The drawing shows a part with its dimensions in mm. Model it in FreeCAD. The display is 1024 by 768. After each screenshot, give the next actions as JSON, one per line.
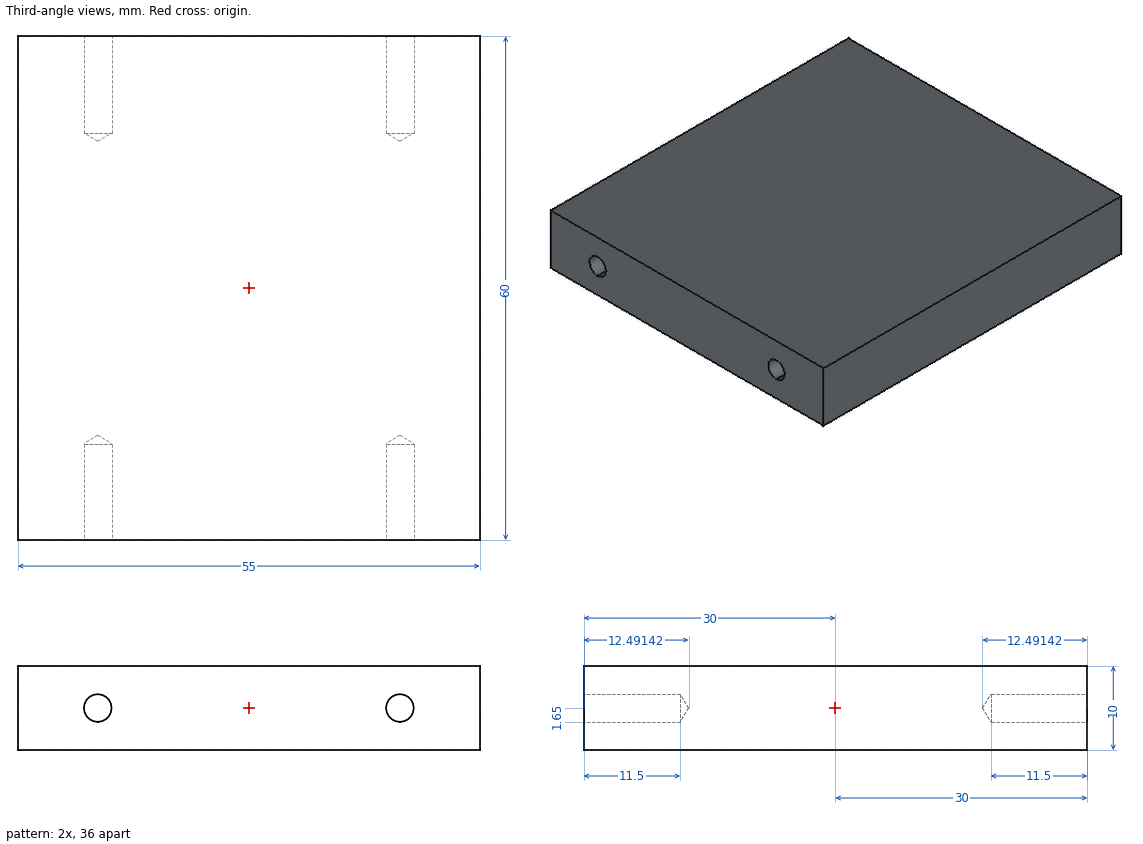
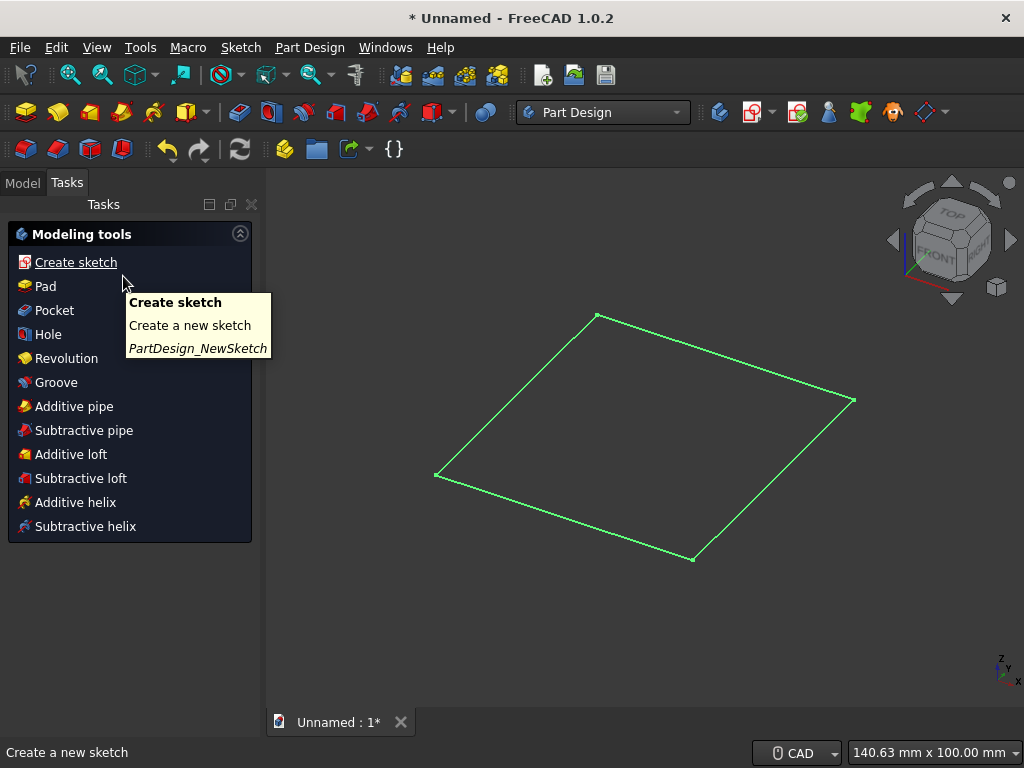
{"action": "left_click", "coordinate": [26, 112]}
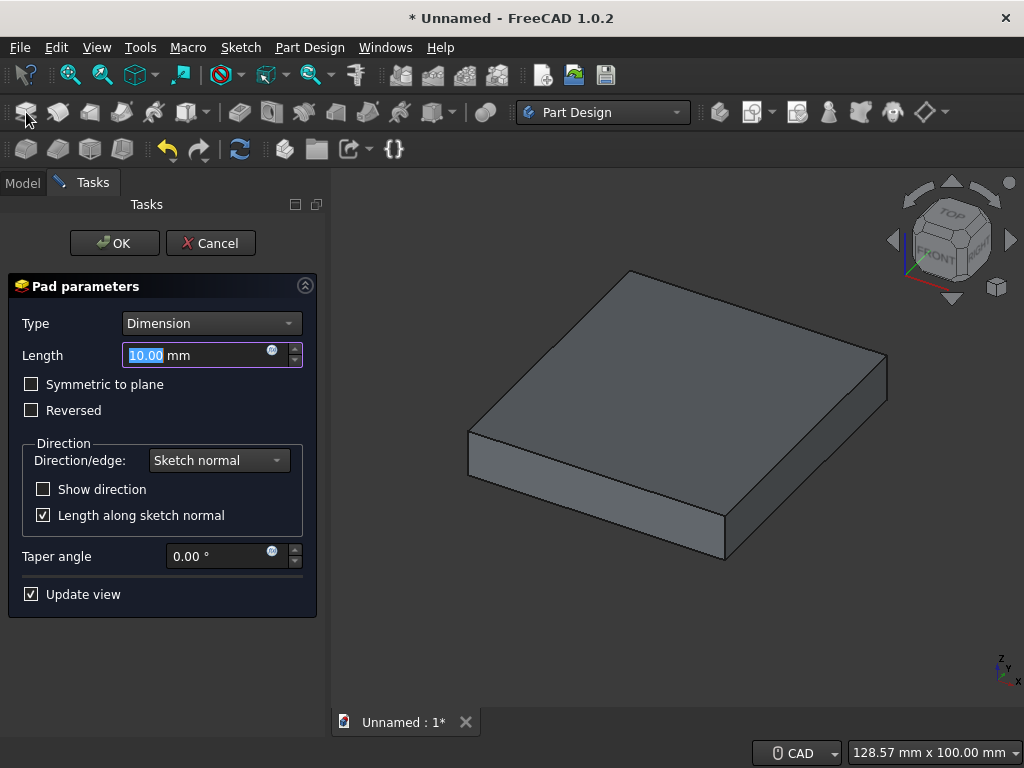
{"action": "type", "text": "10"}
{"action": "key", "text": "Tab"}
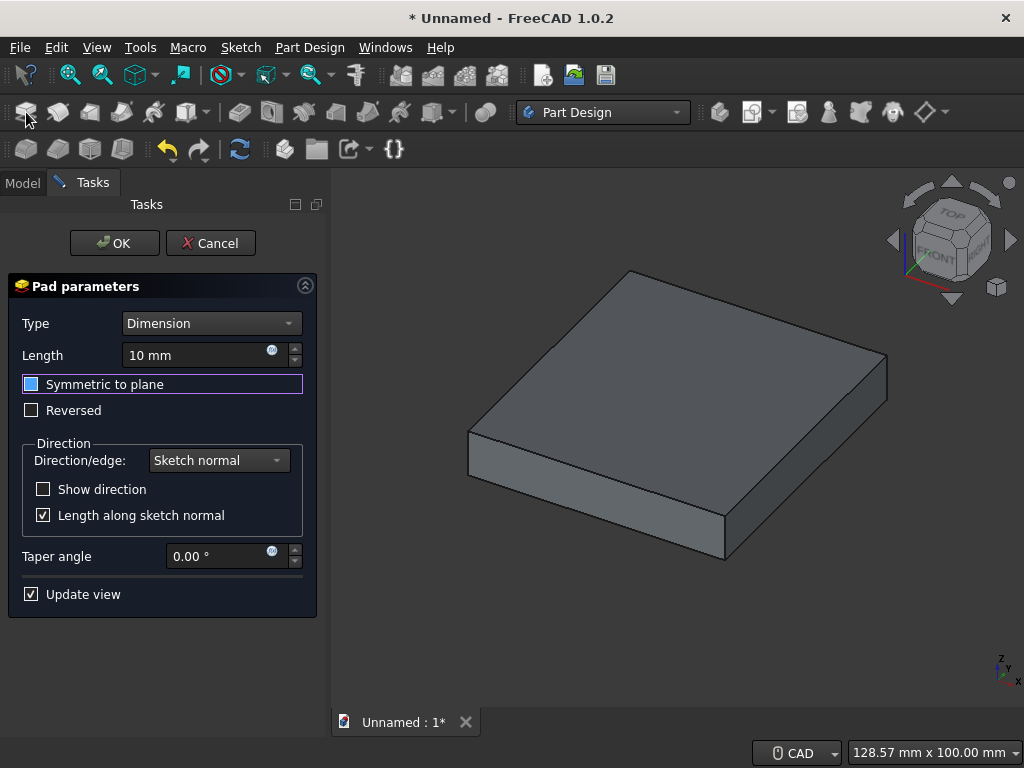
{"action": "left_click", "coordinate": [30, 384]}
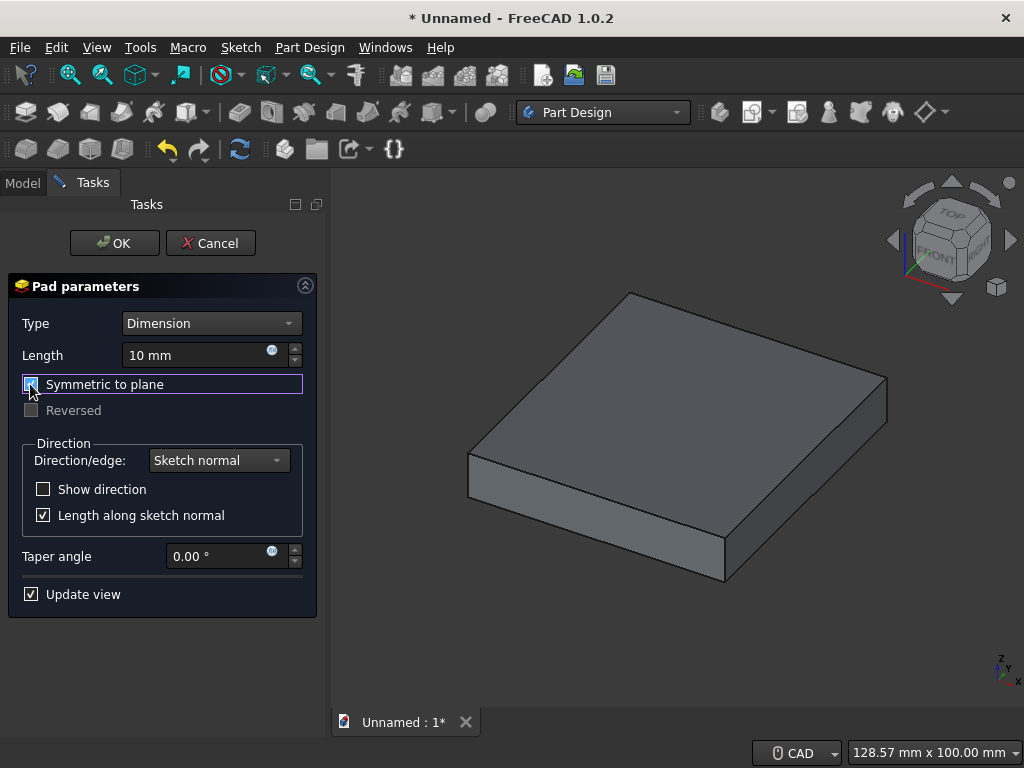
{"action": "left_click", "coordinate": [115, 243]}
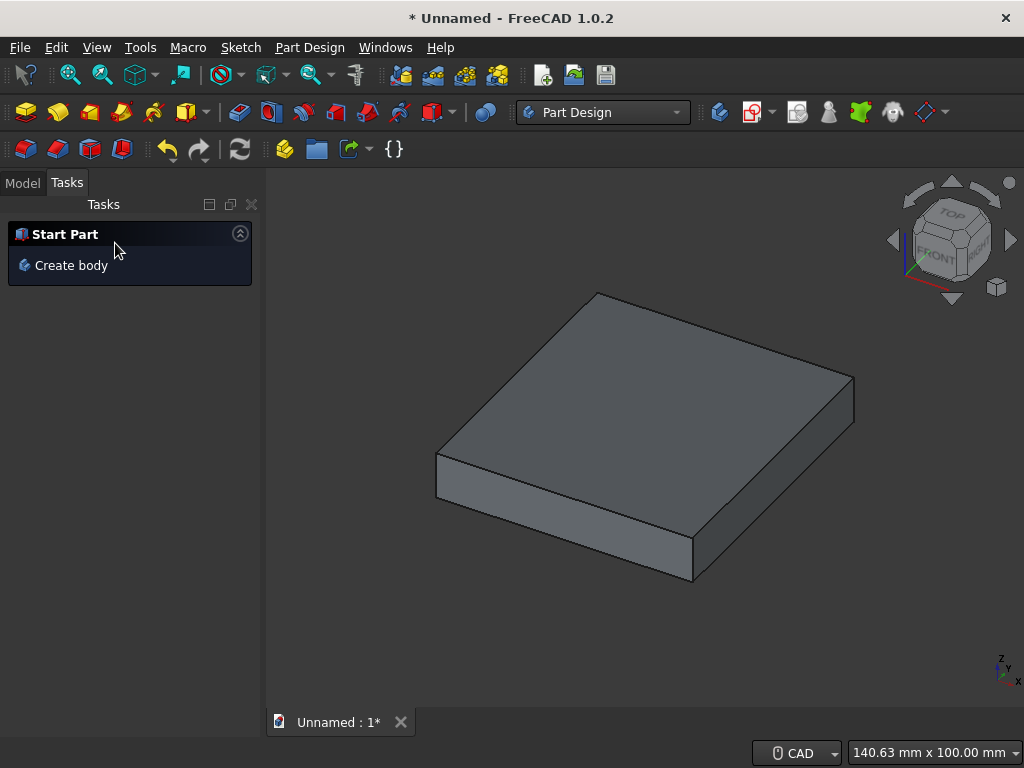
{"action": "left_click", "coordinate": [23, 182]}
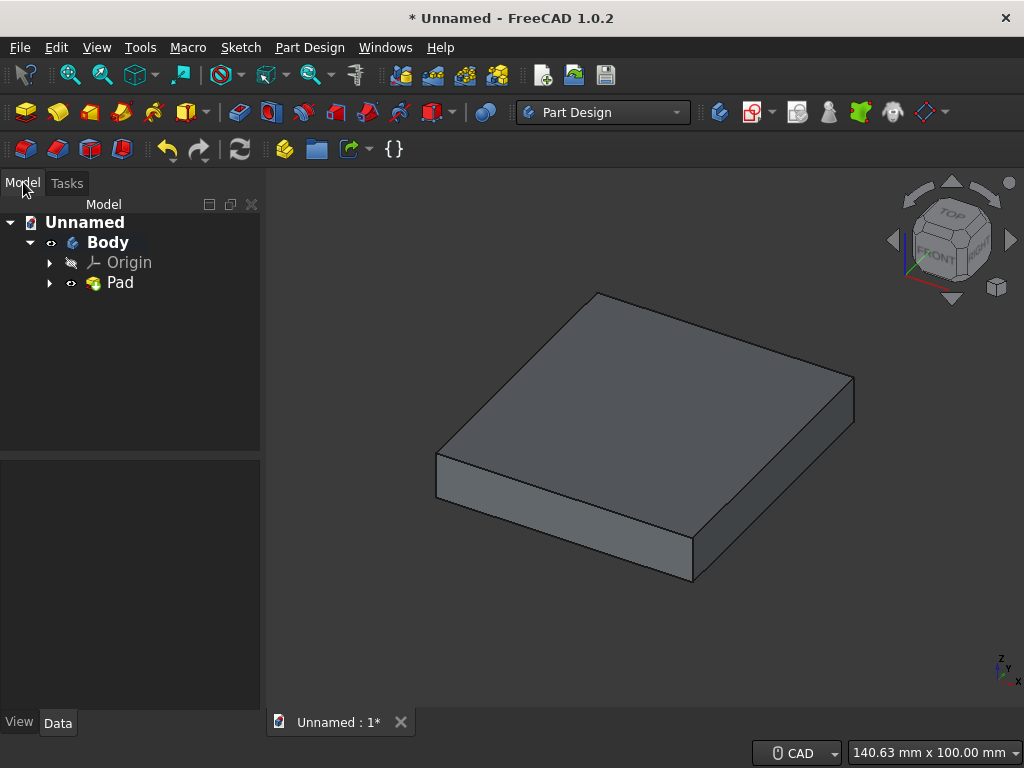
{"action": "left_click", "coordinate": [50, 263]}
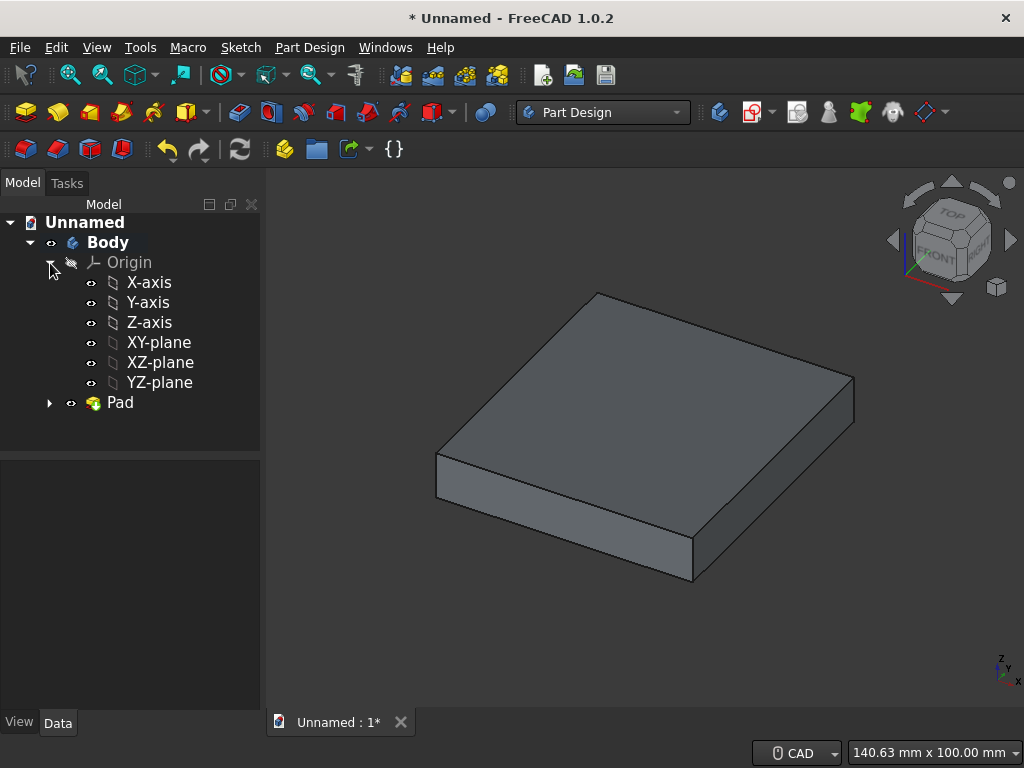
{"action": "left_click", "coordinate": [136, 383]}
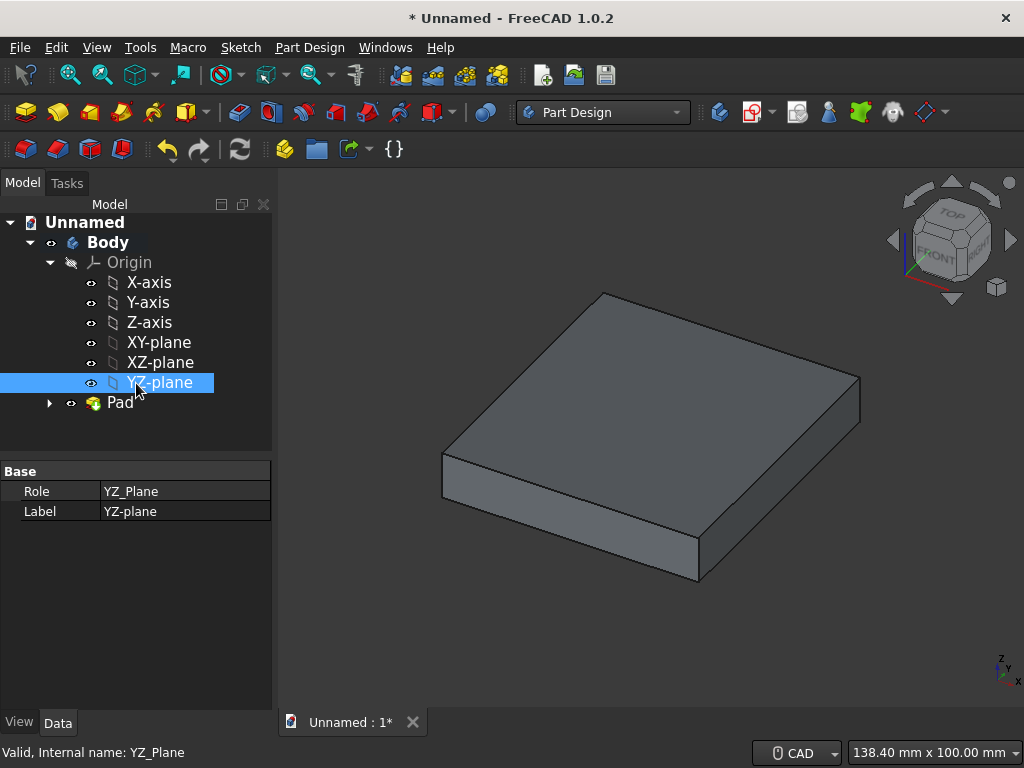
{"action": "left_click", "coordinate": [926, 112]}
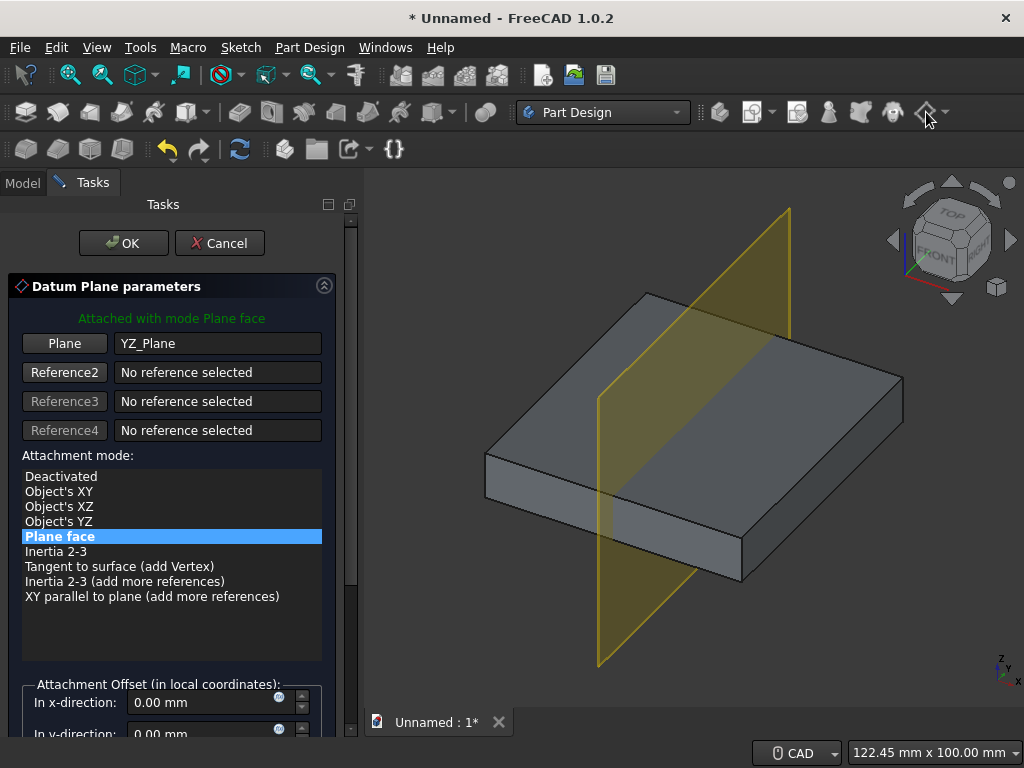
{"action": "scroll", "coordinate": [351, 475], "scroll_direction": "down", "scroll_amount": 2}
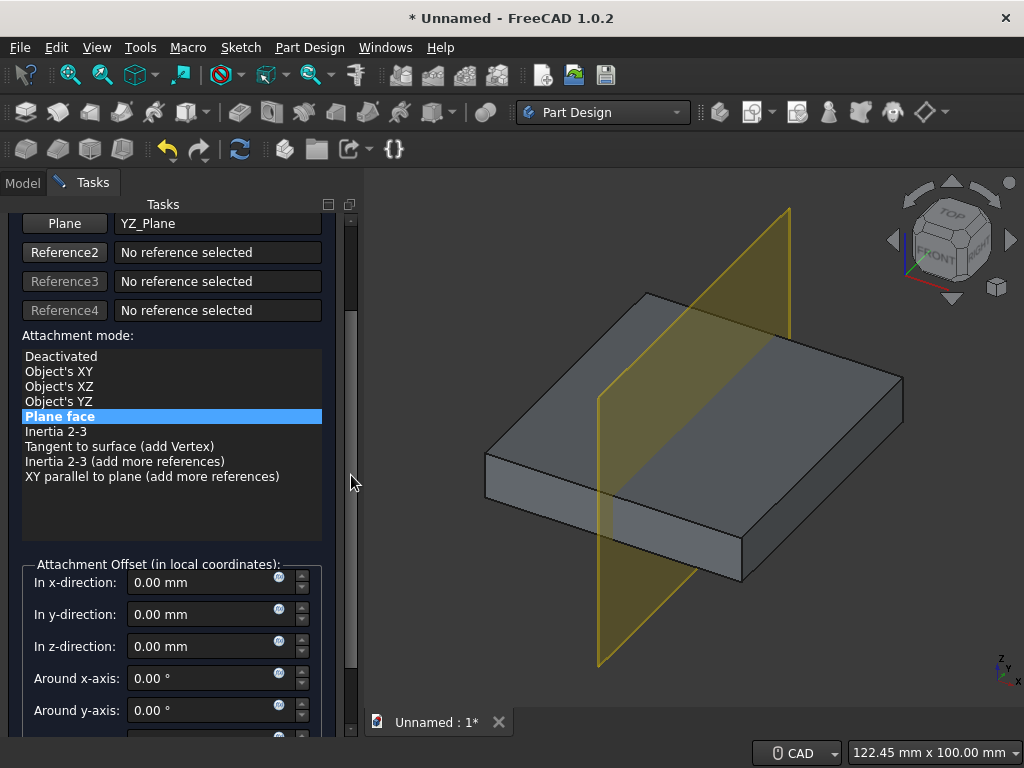
{"action": "triple_click", "coordinate": [210, 646]}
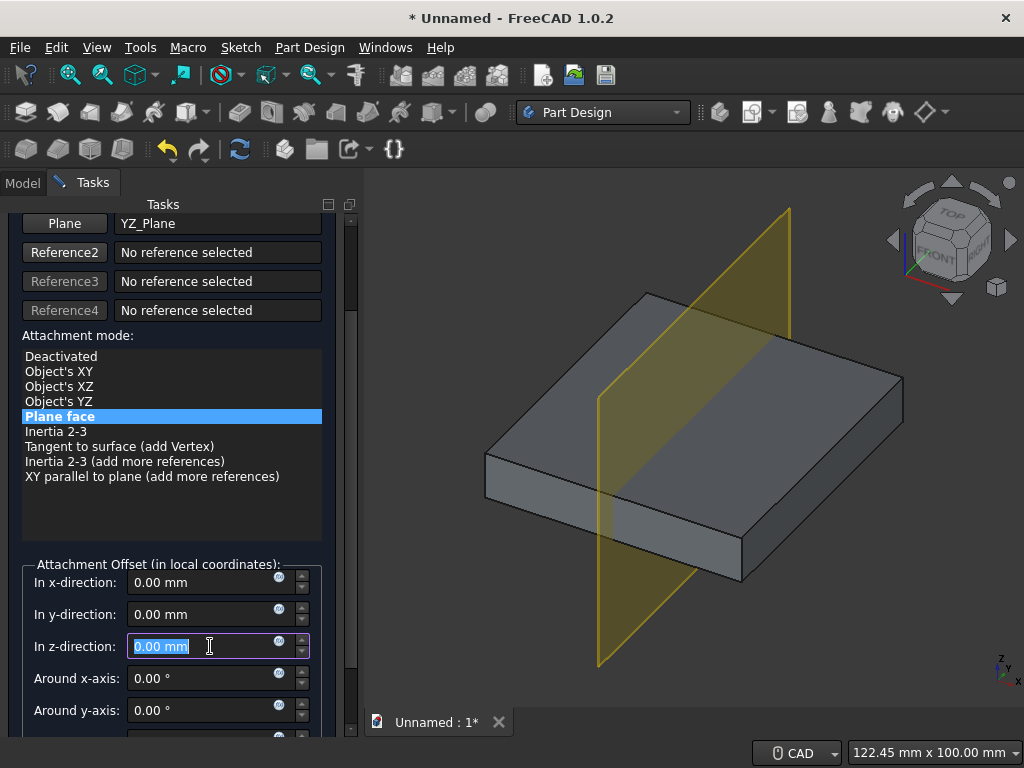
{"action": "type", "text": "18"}
{"action": "key", "text": "Tab"}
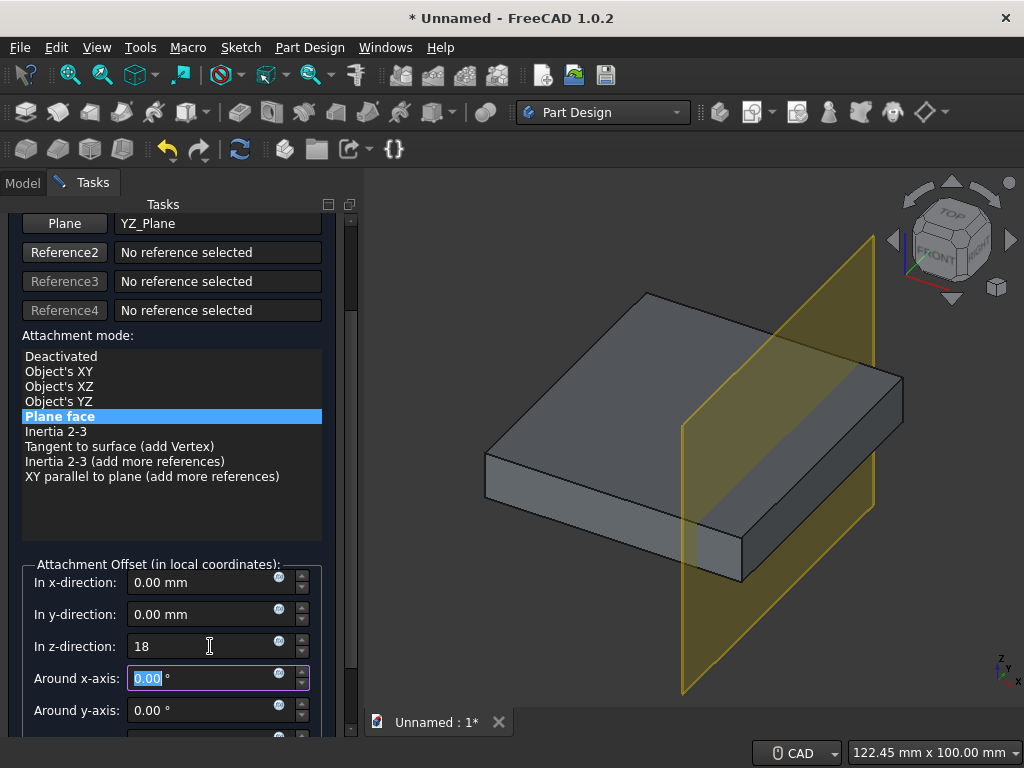
{"action": "scroll", "coordinate": [351, 475], "scroll_direction": "up", "scroll_amount": 3}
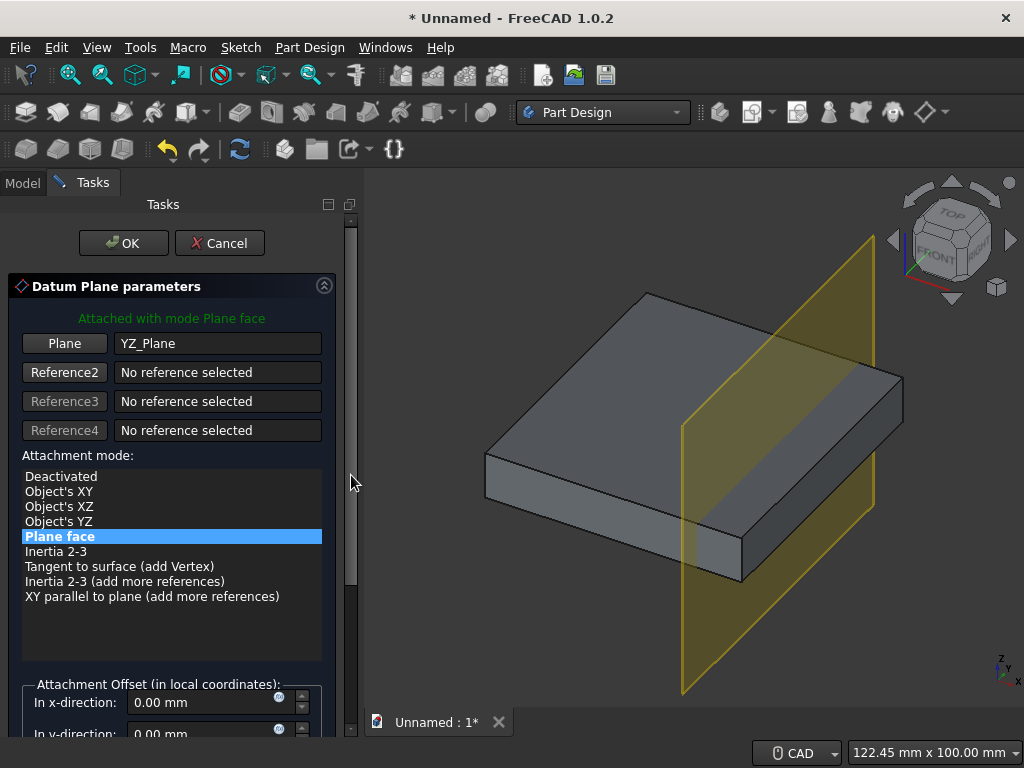
{"action": "left_click", "coordinate": [124, 243]}